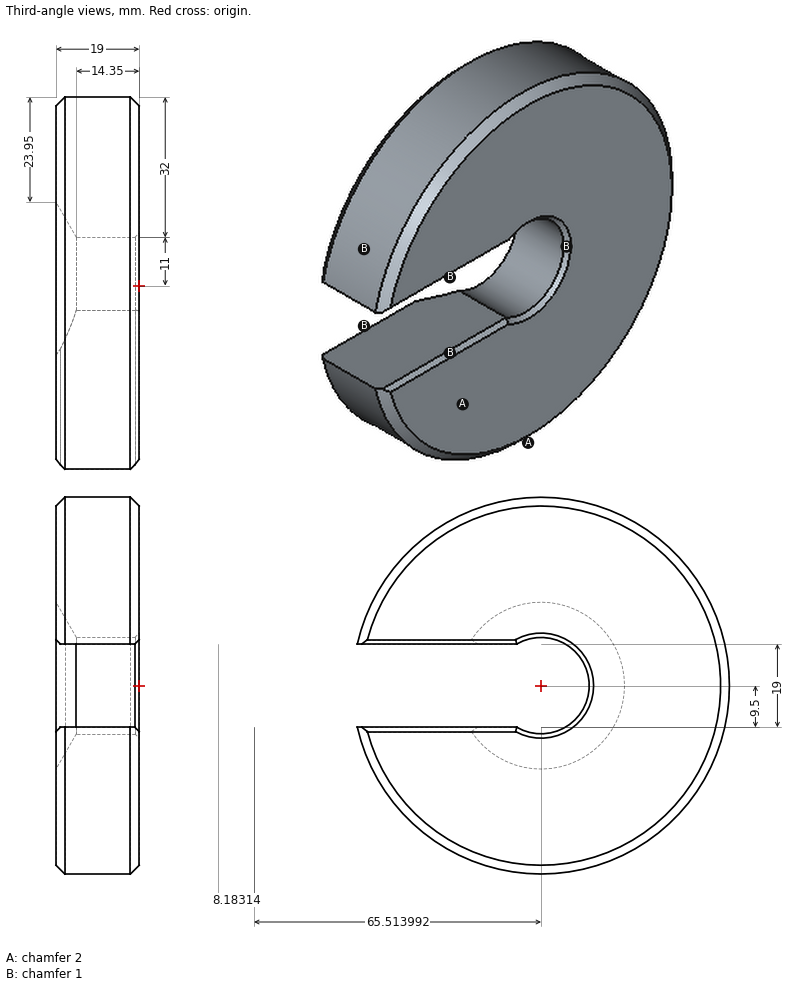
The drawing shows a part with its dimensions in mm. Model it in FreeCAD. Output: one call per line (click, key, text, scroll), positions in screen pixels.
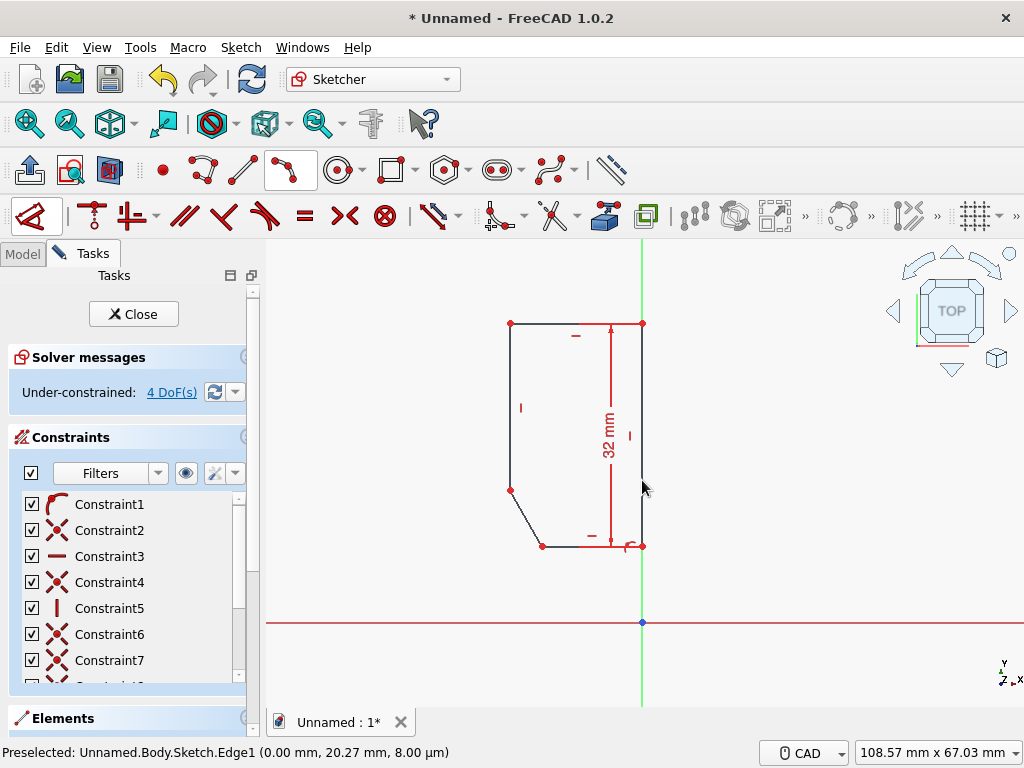
click(603, 324)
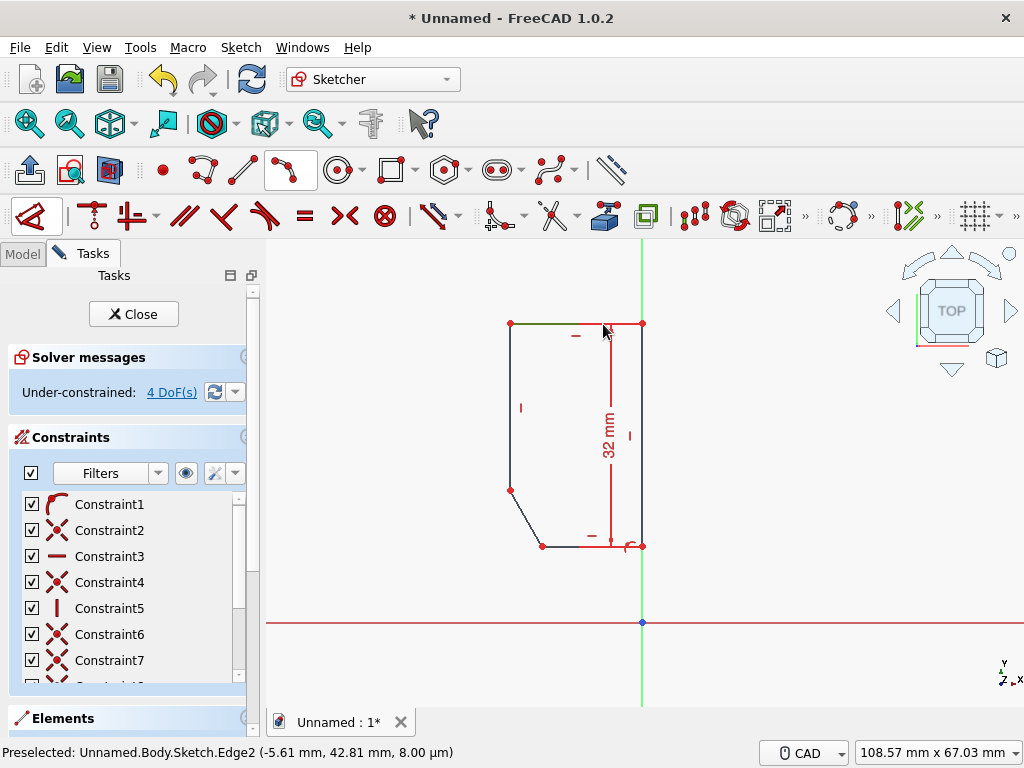
key(l)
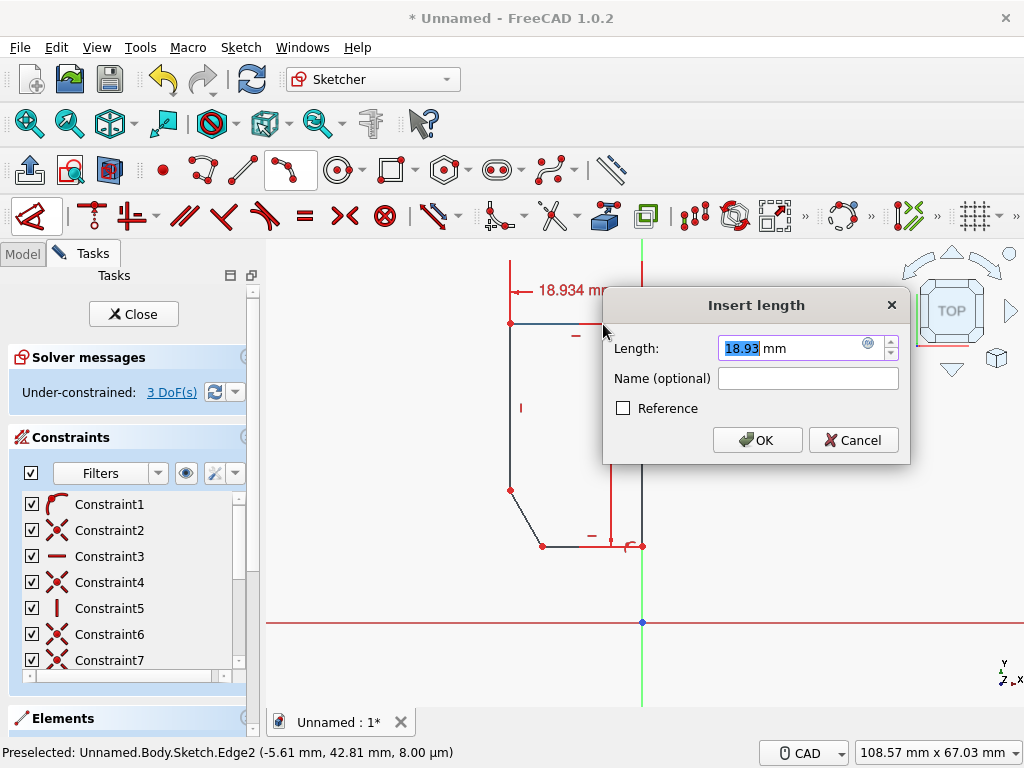
text(19)
key(Return)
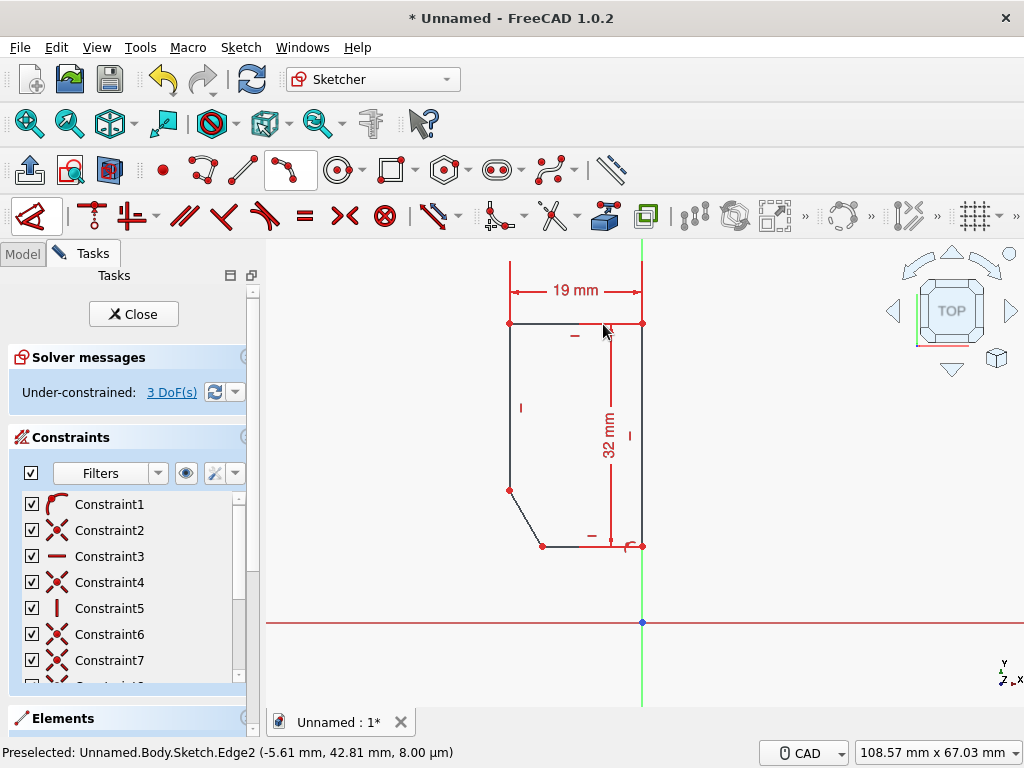
click(642, 547)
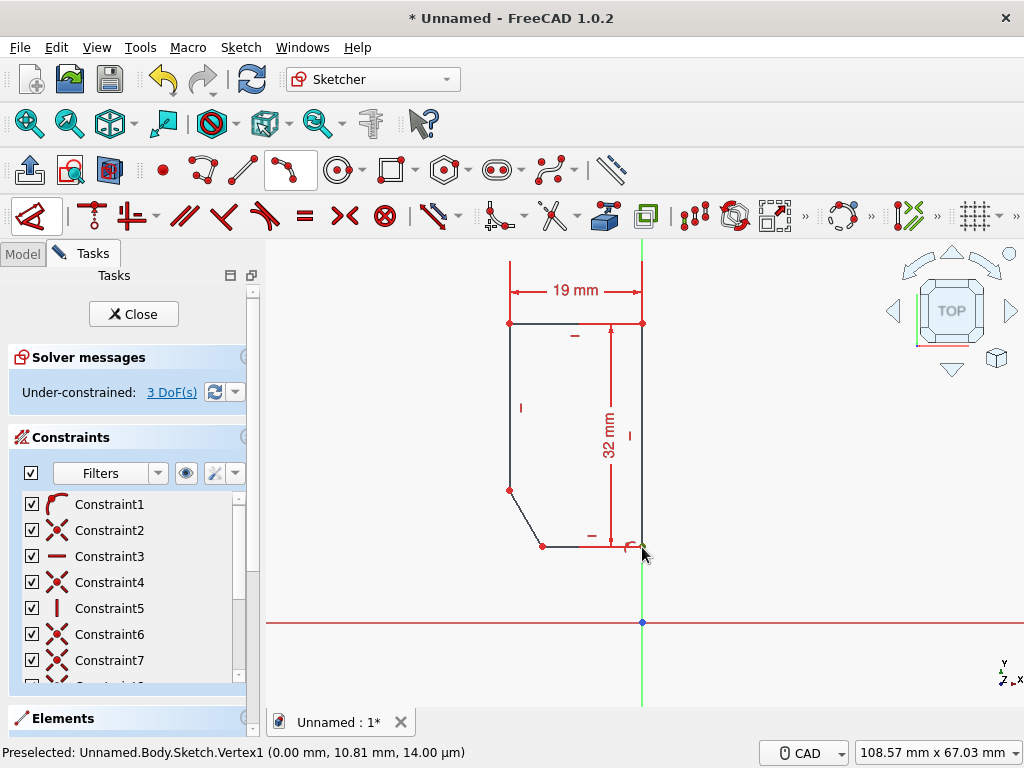
click(56, 216)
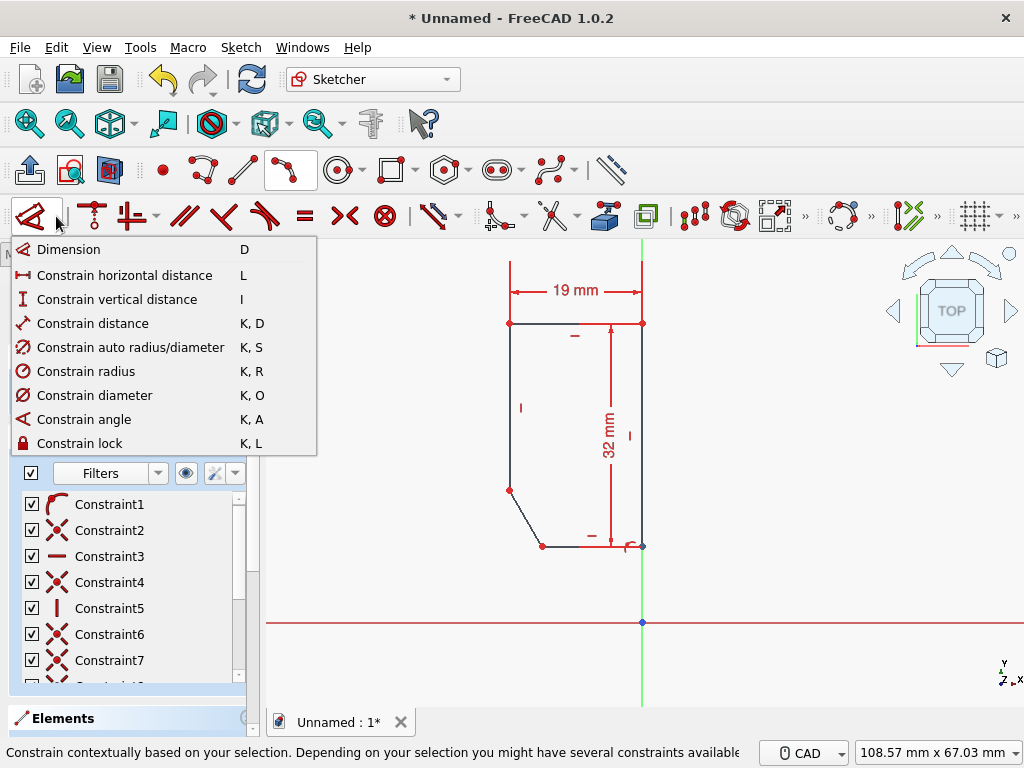
click(164, 299)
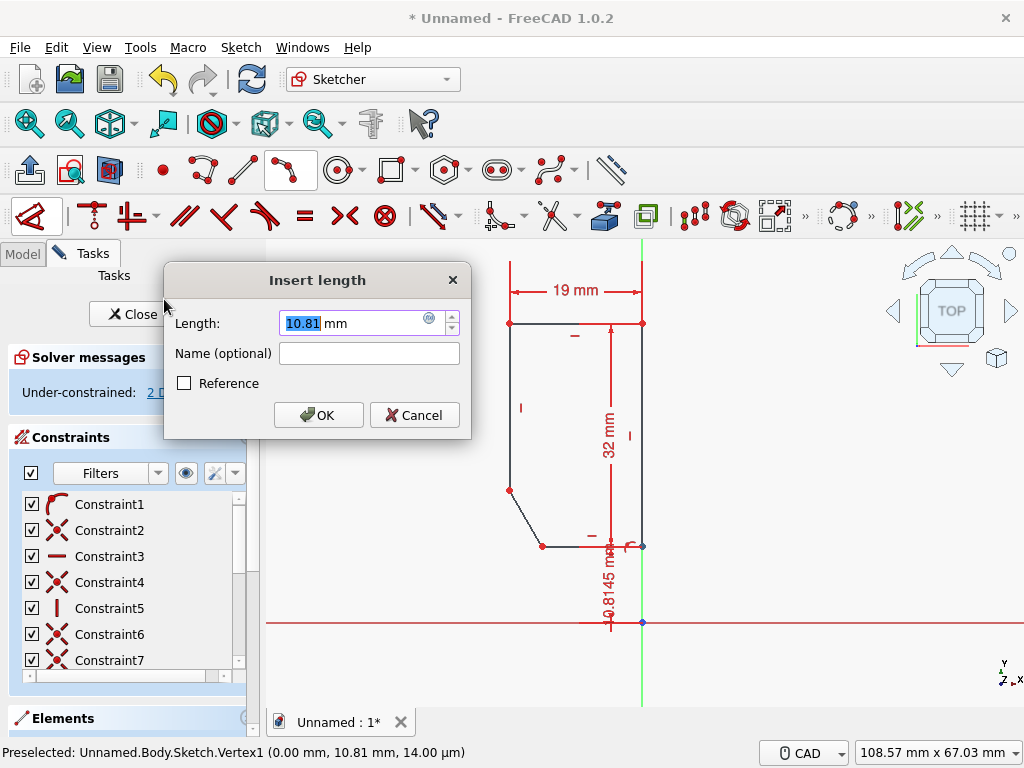
text(11)
key(Return)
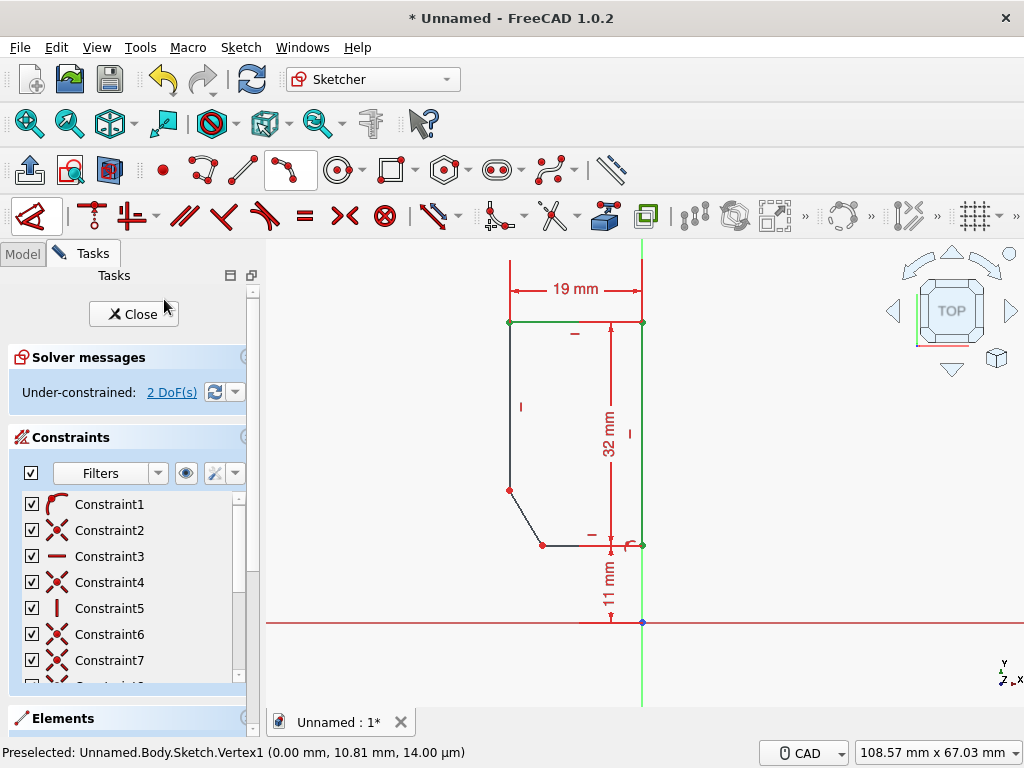
click(510, 373)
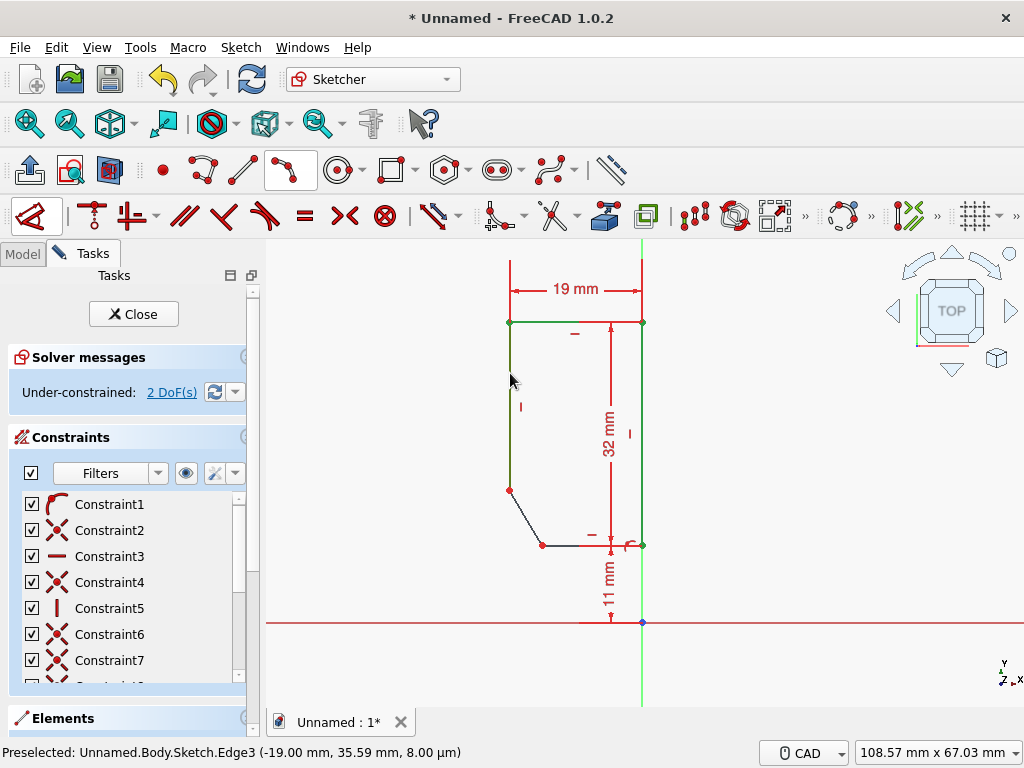
click(56, 216)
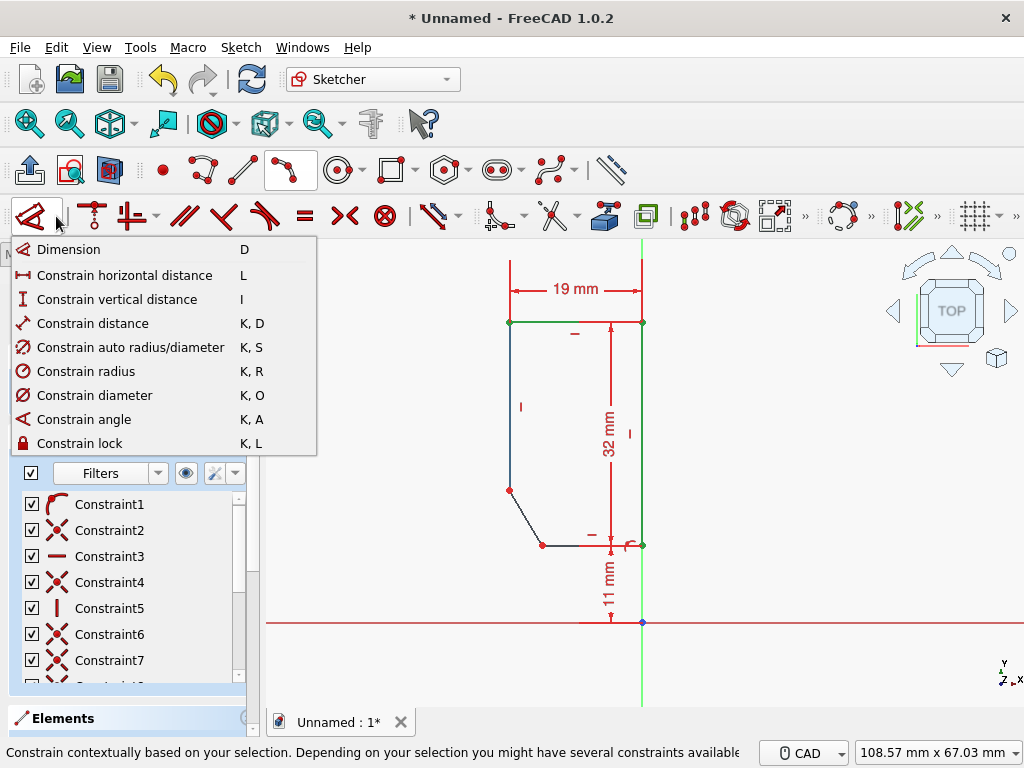
click(164, 299)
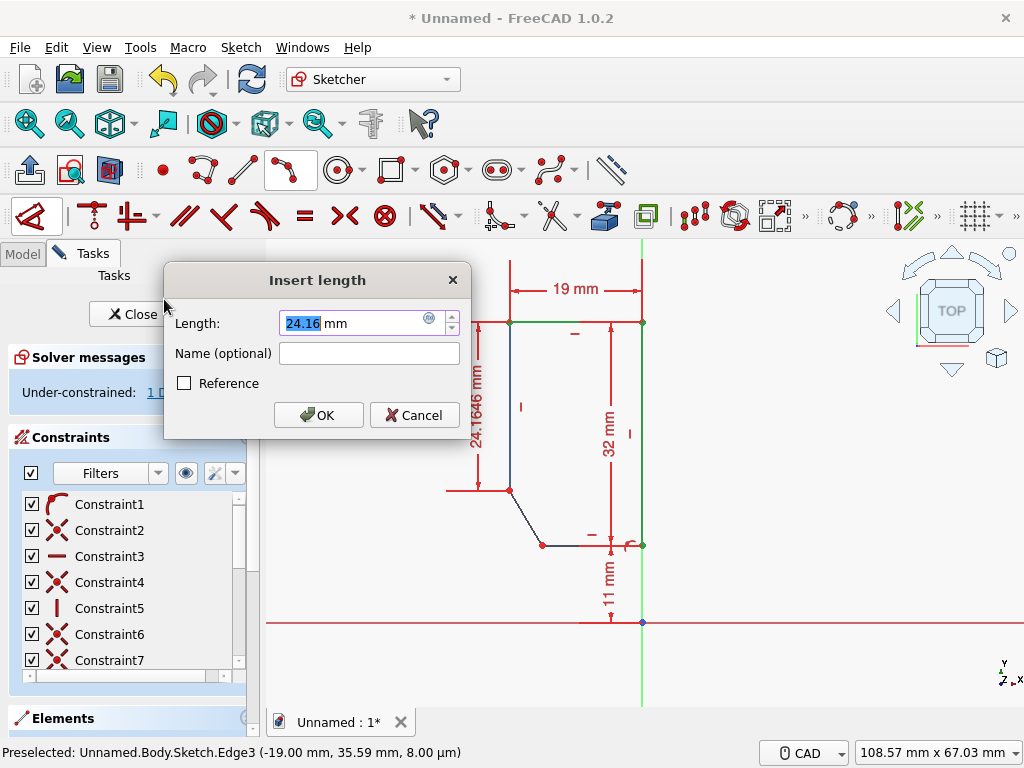
text(23.95)
key(Return)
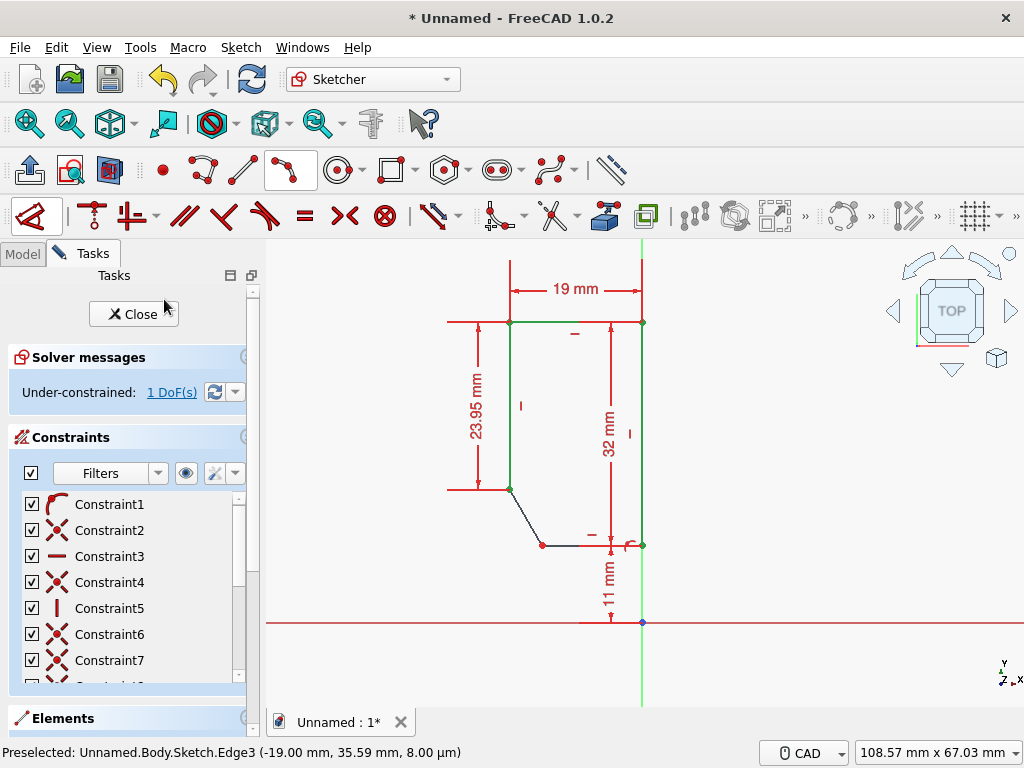
click(572, 546)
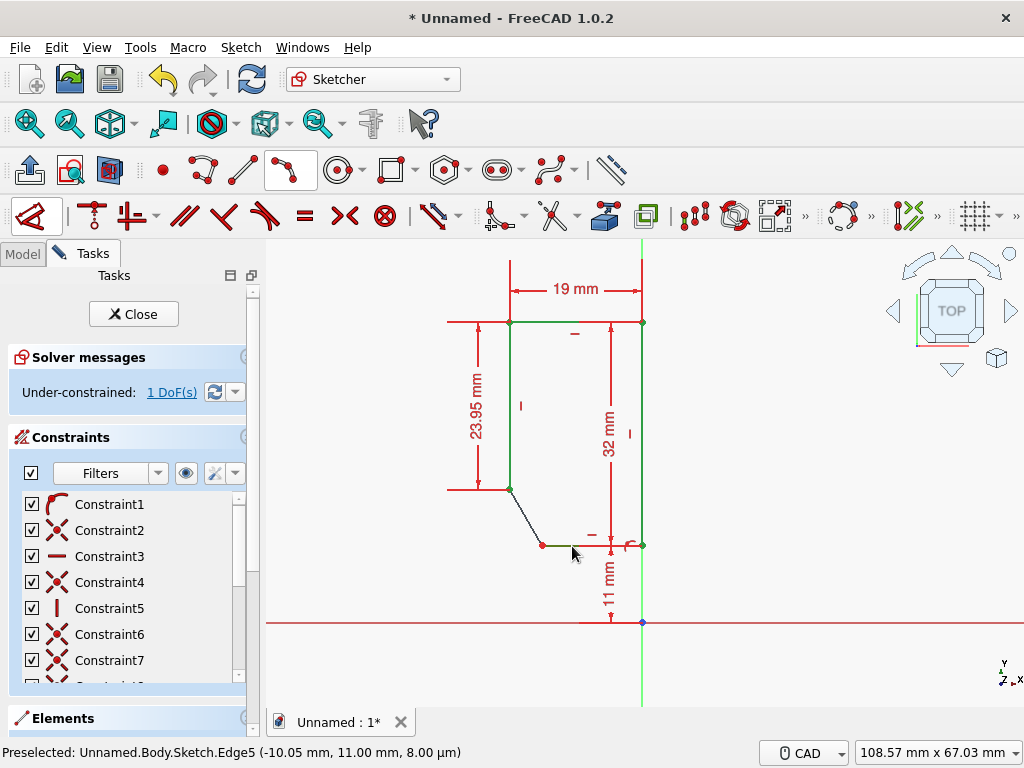
key(l)